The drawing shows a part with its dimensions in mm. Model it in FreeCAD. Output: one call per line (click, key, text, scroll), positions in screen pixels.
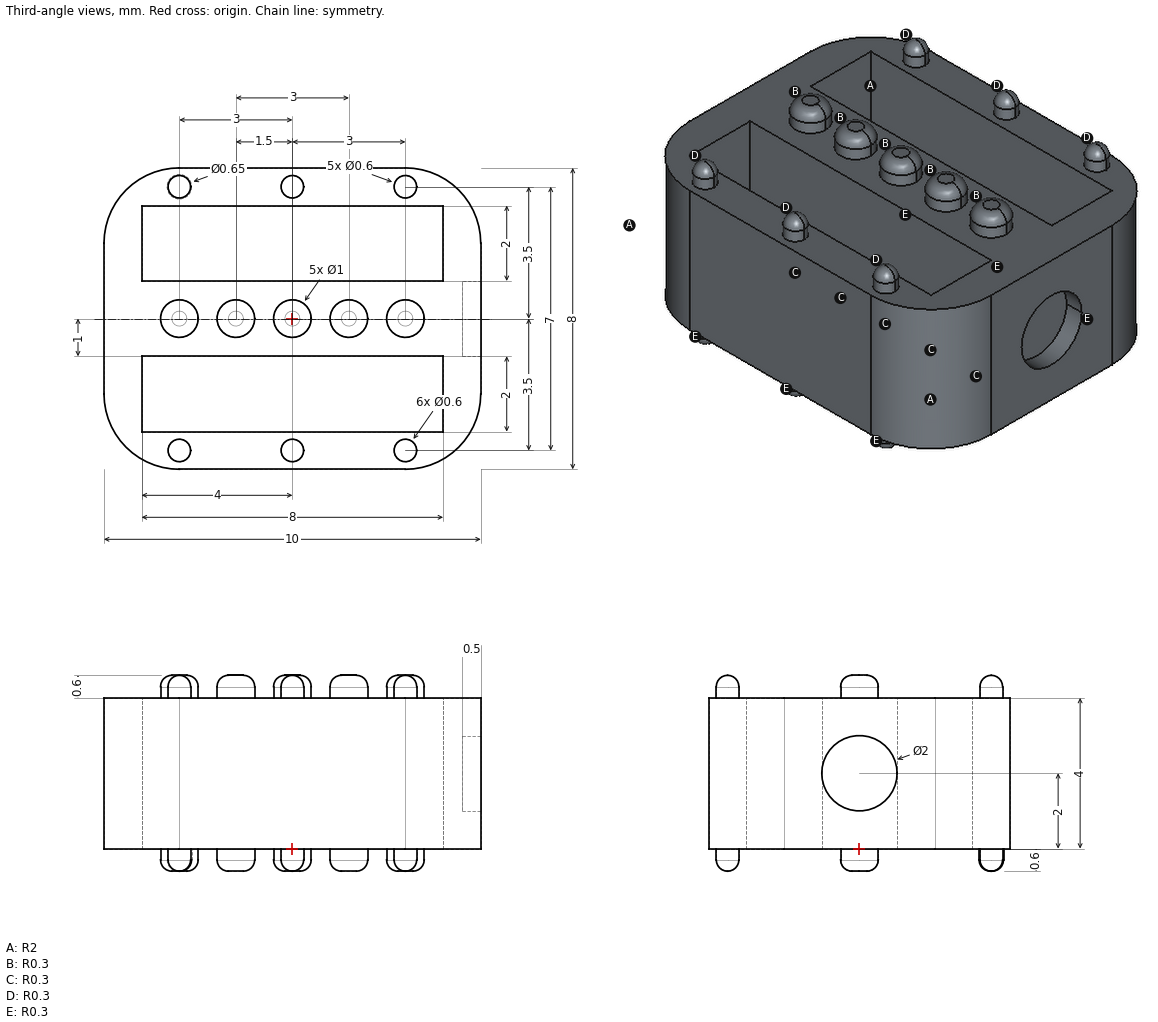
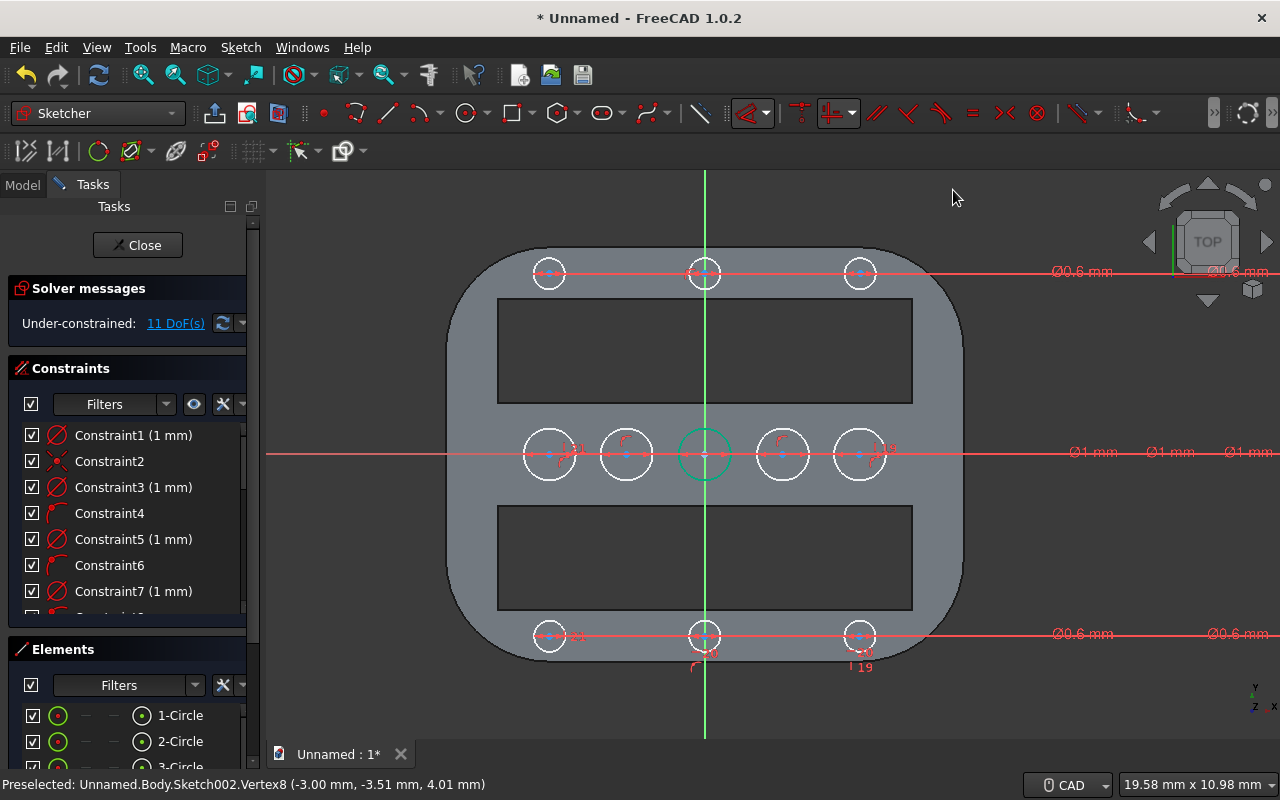
click(705, 636)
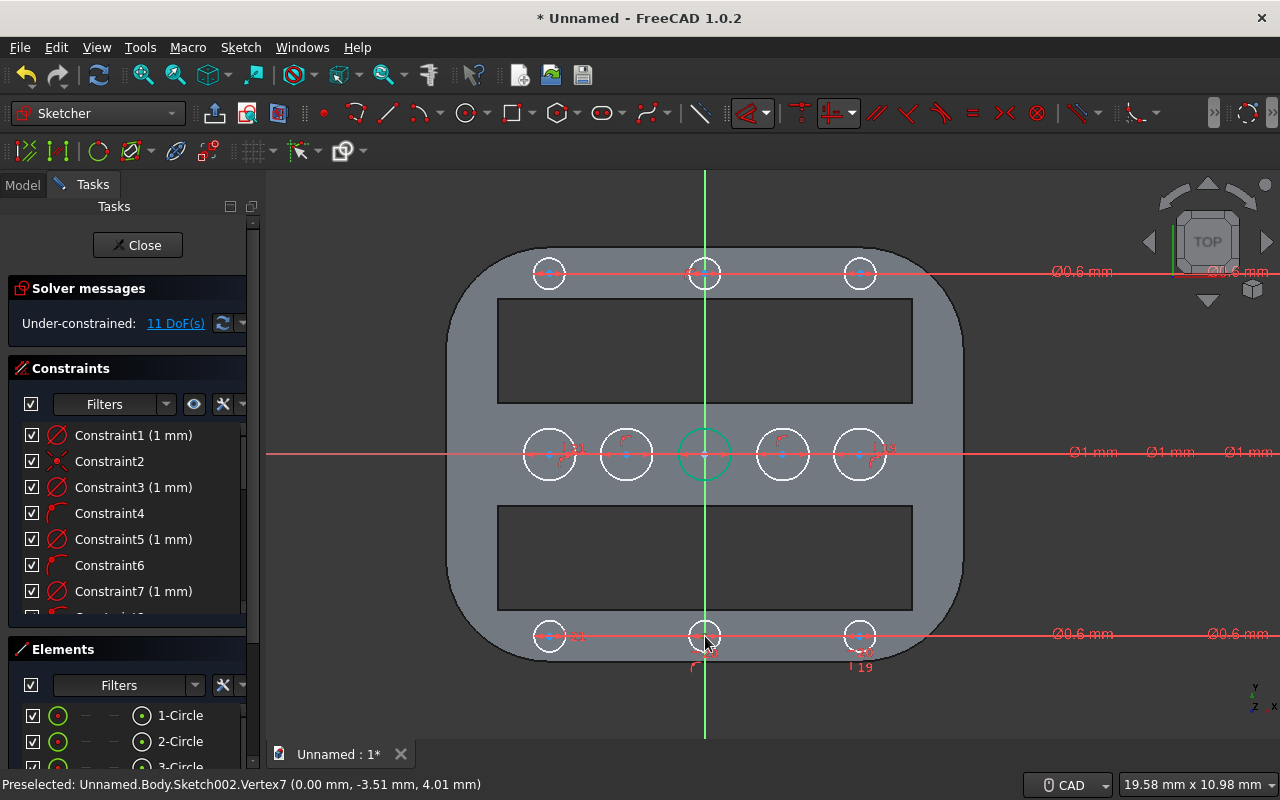
click(550, 636)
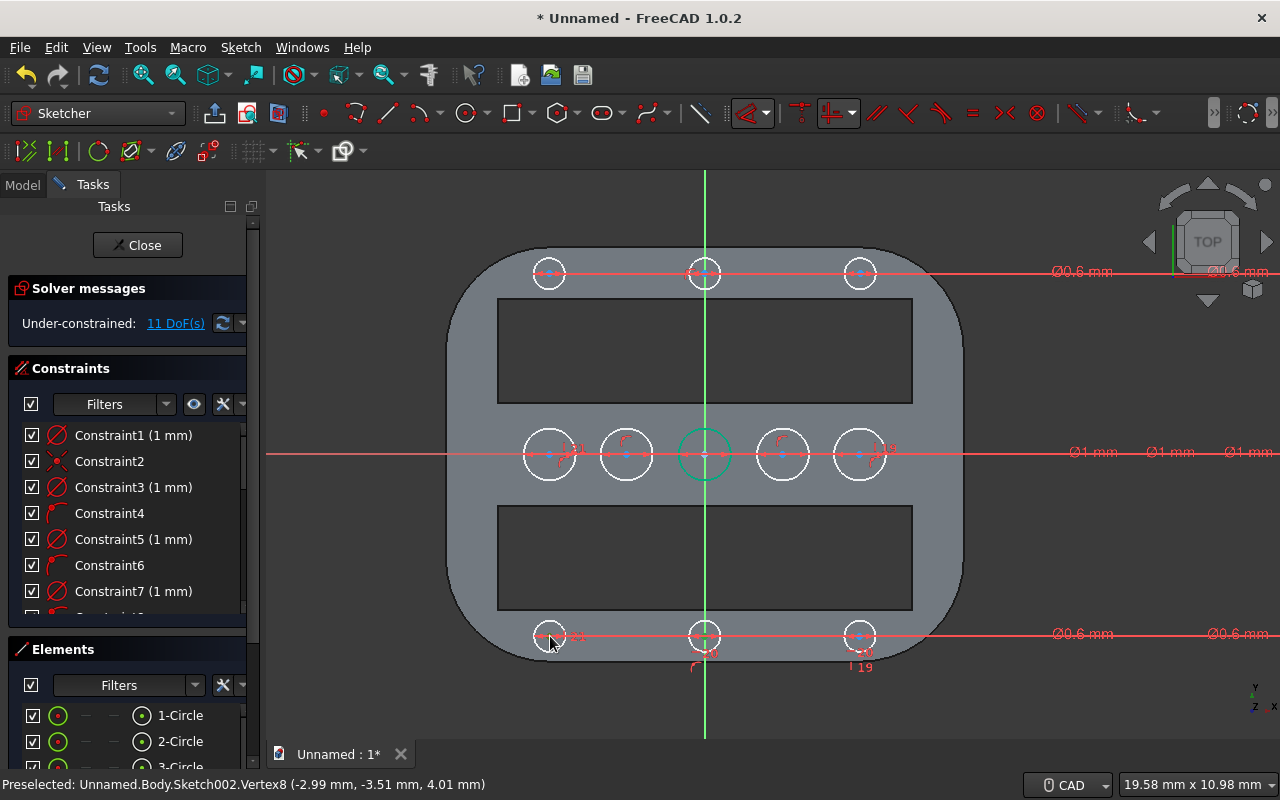
key(h)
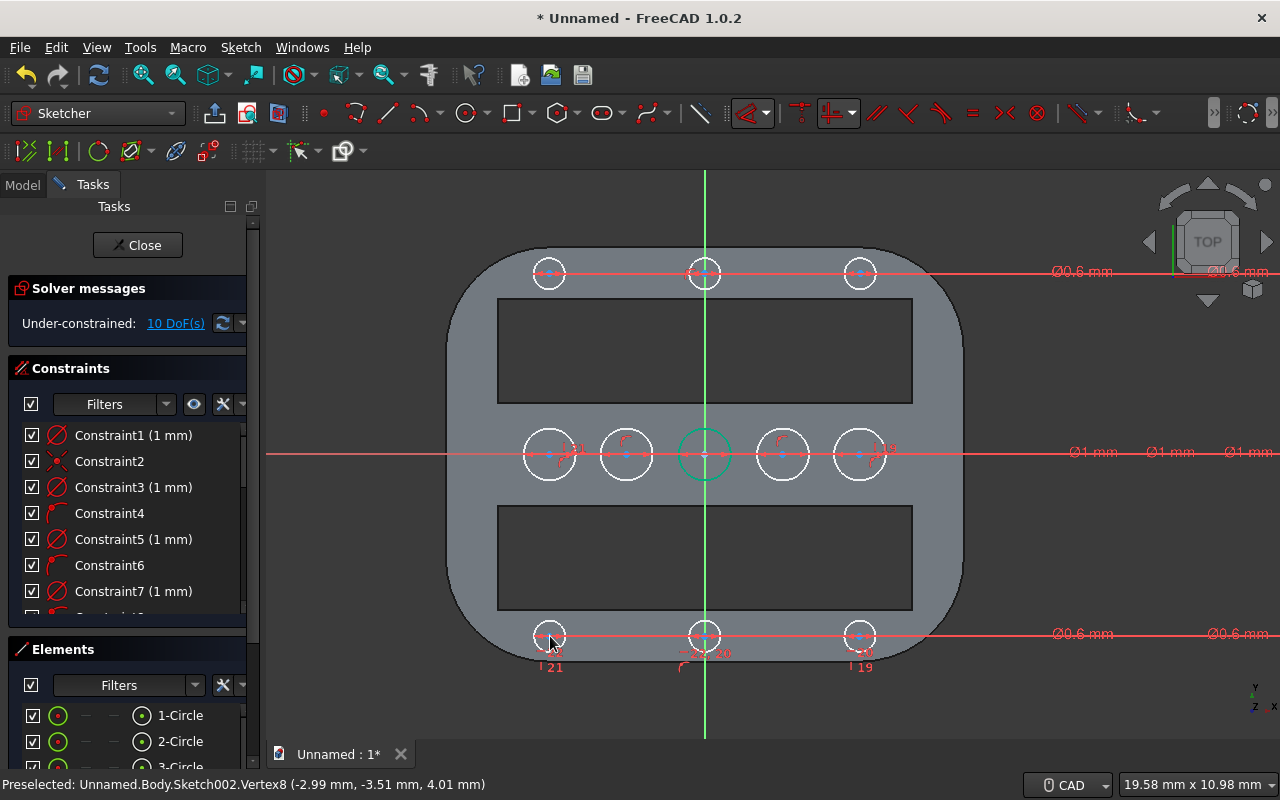
click(860, 454)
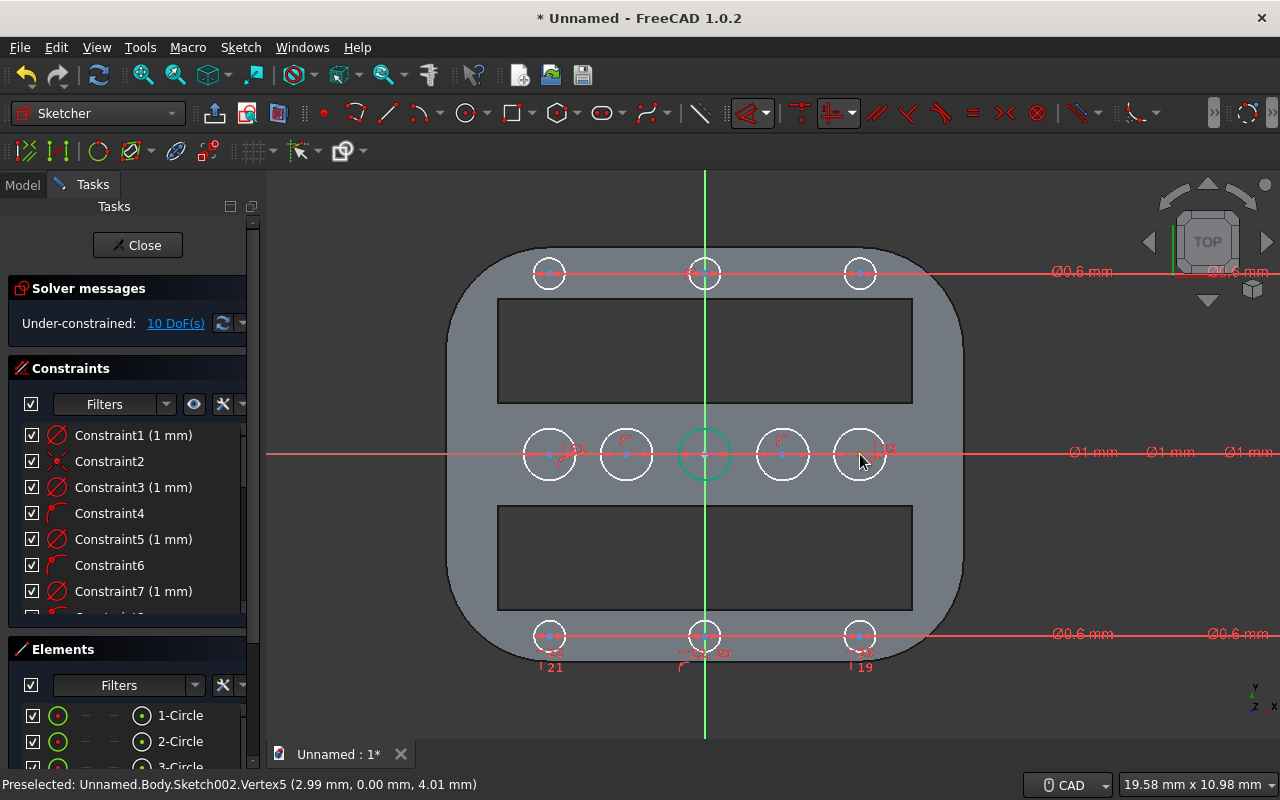
click(860, 274)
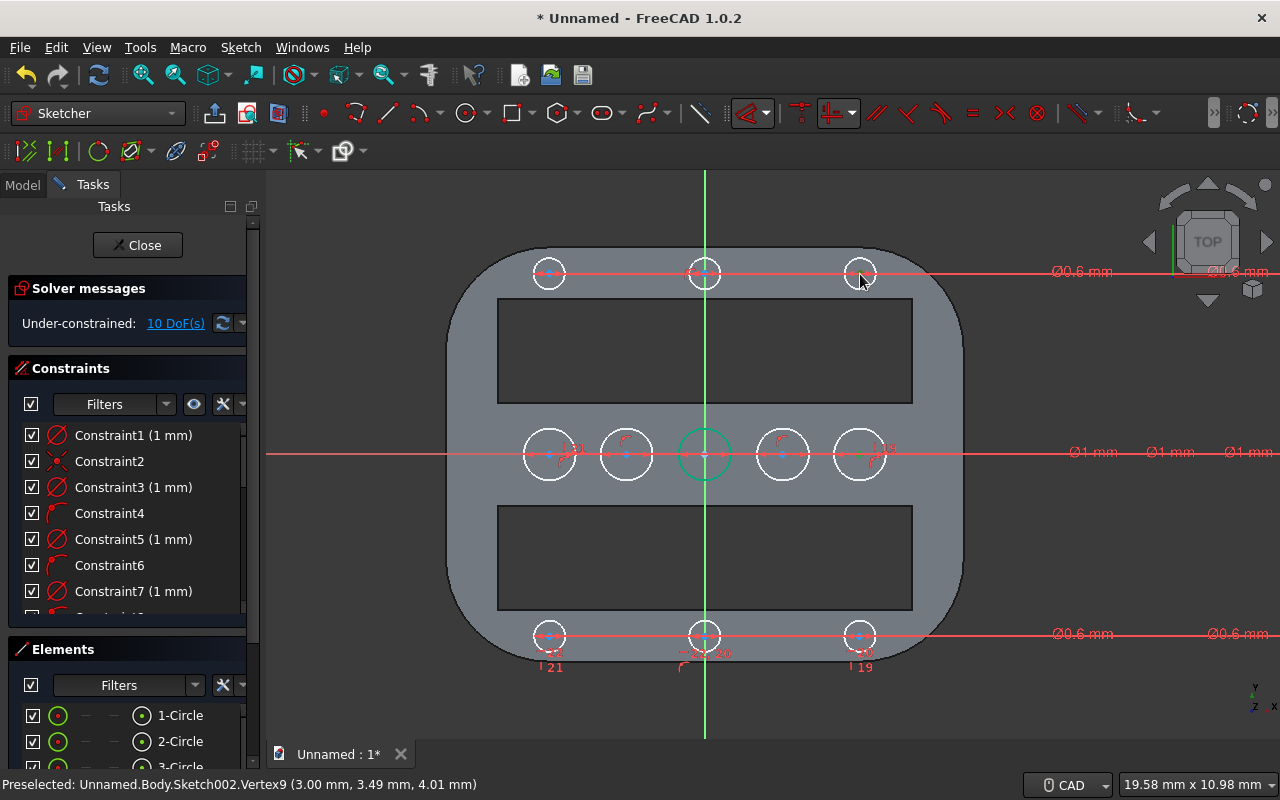
click(854, 114)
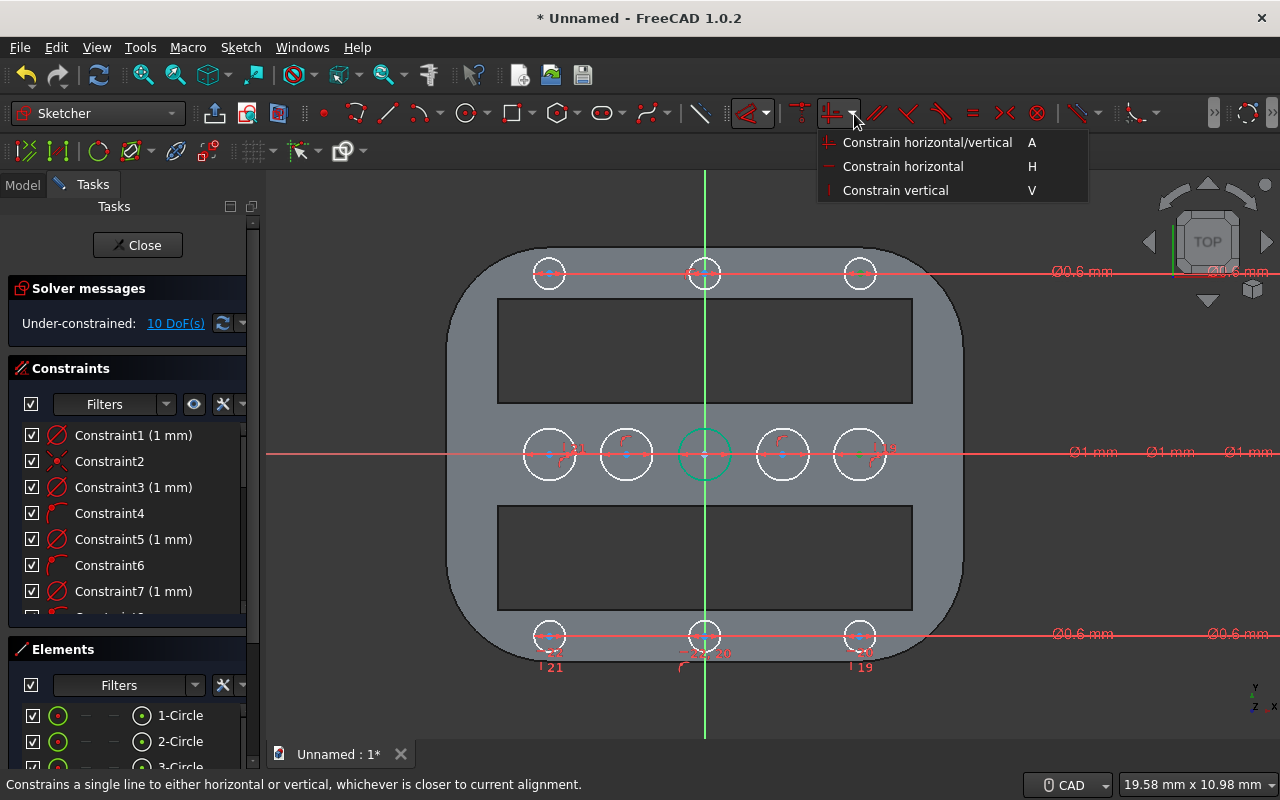
click(953, 190)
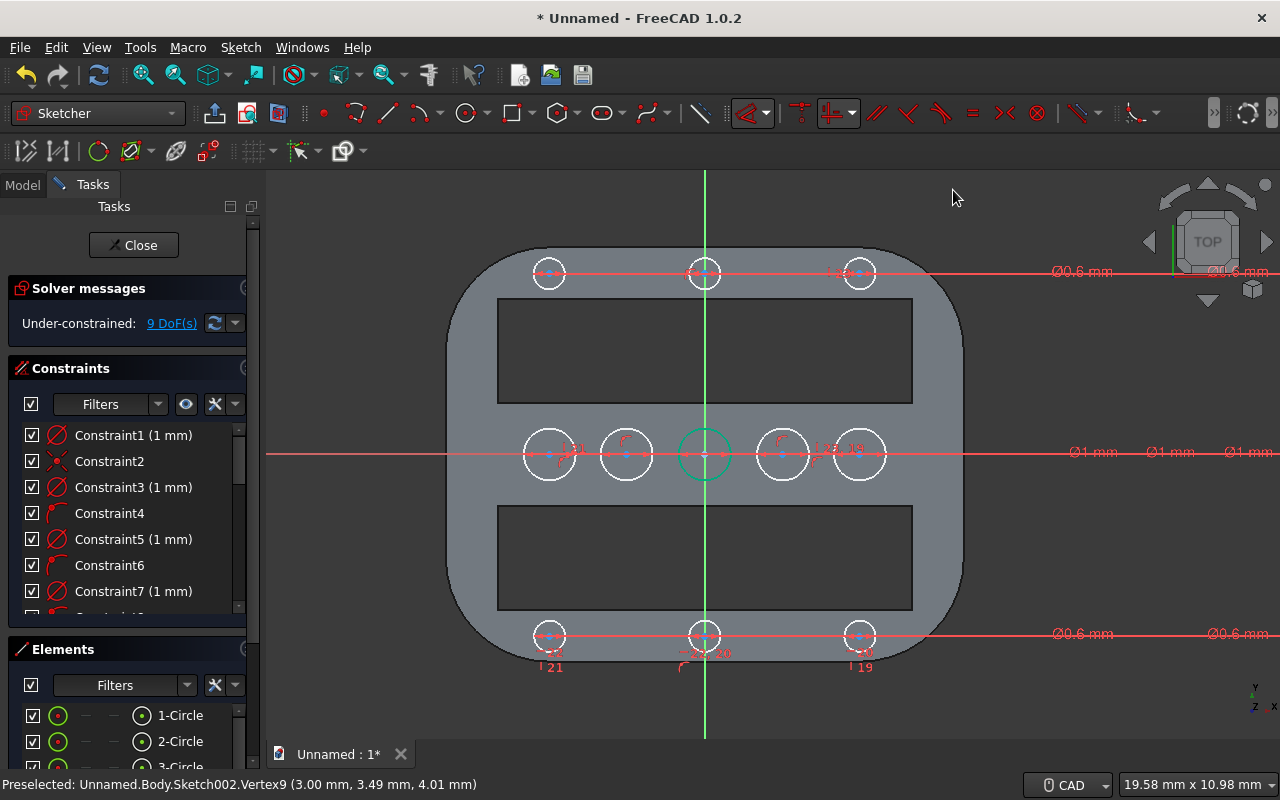
click(860, 274)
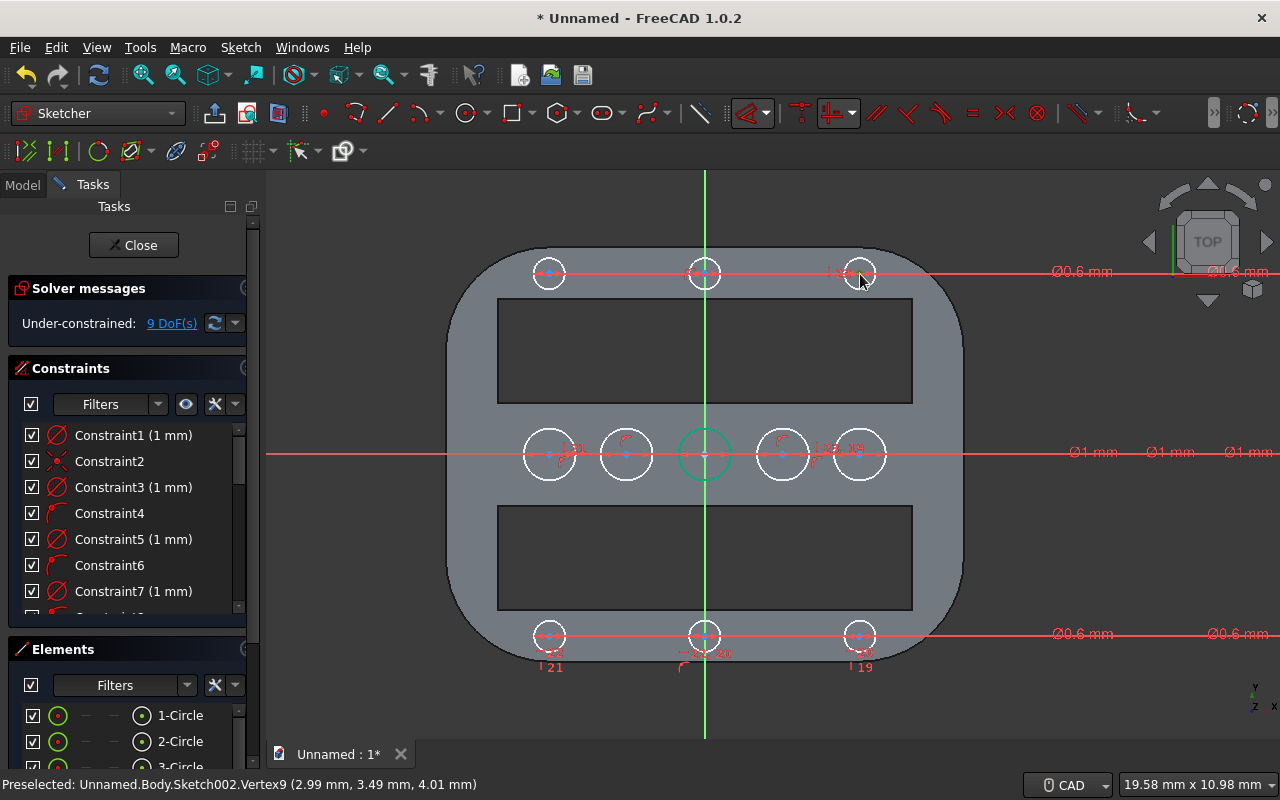
click(705, 274)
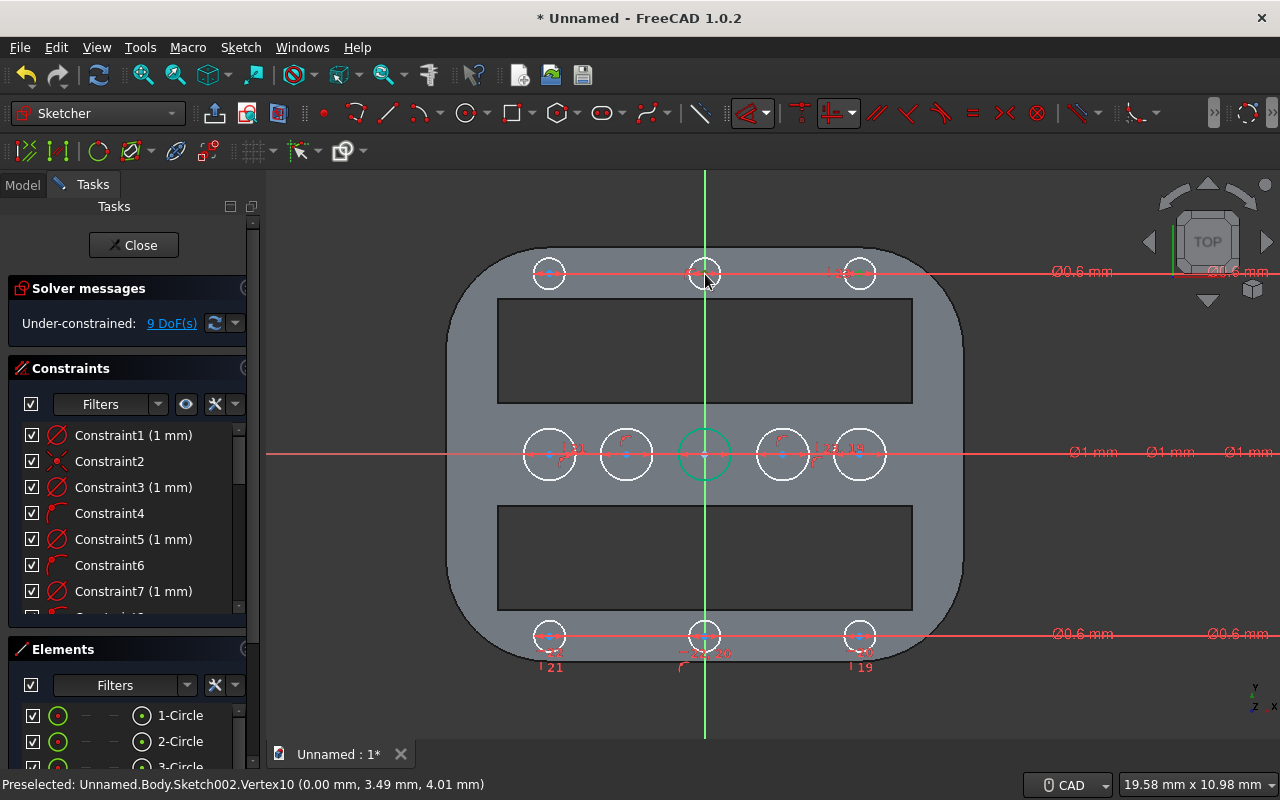
click(854, 114)